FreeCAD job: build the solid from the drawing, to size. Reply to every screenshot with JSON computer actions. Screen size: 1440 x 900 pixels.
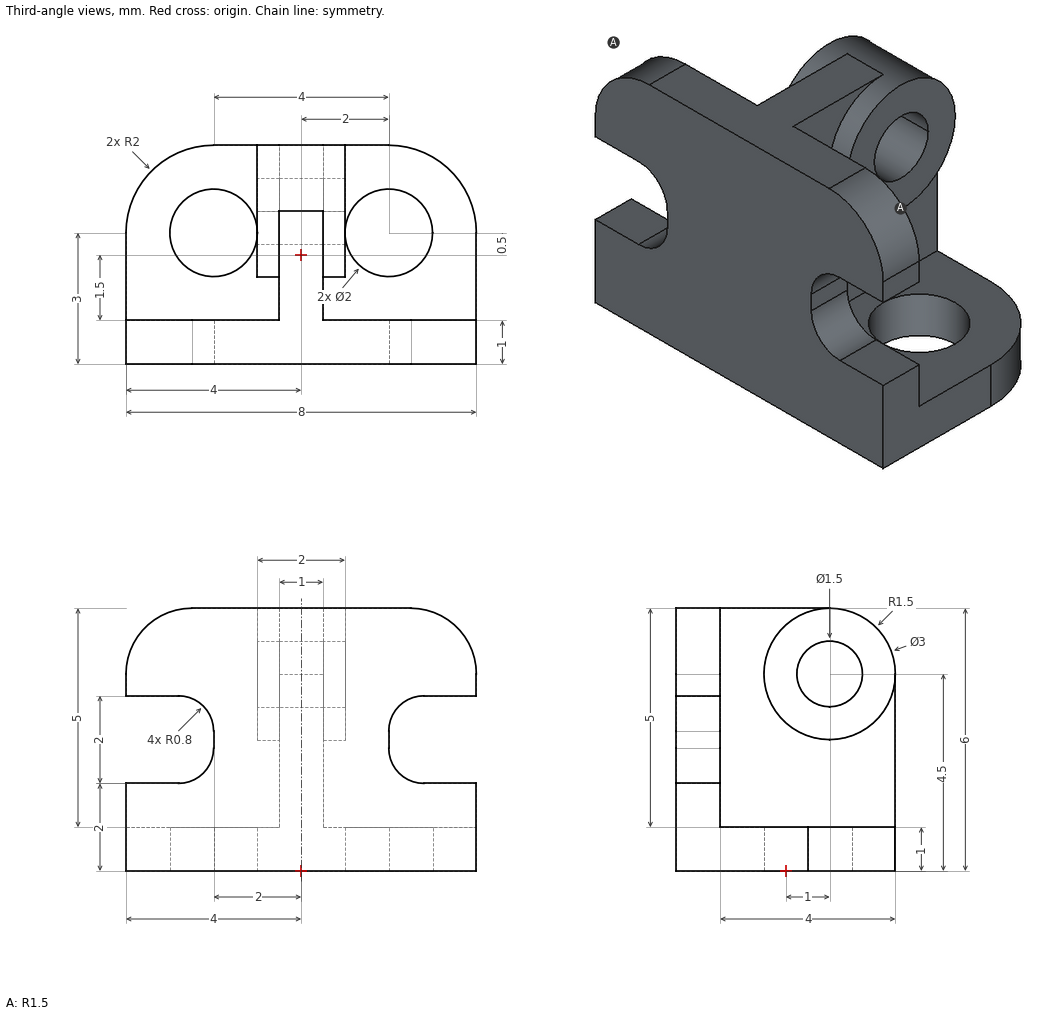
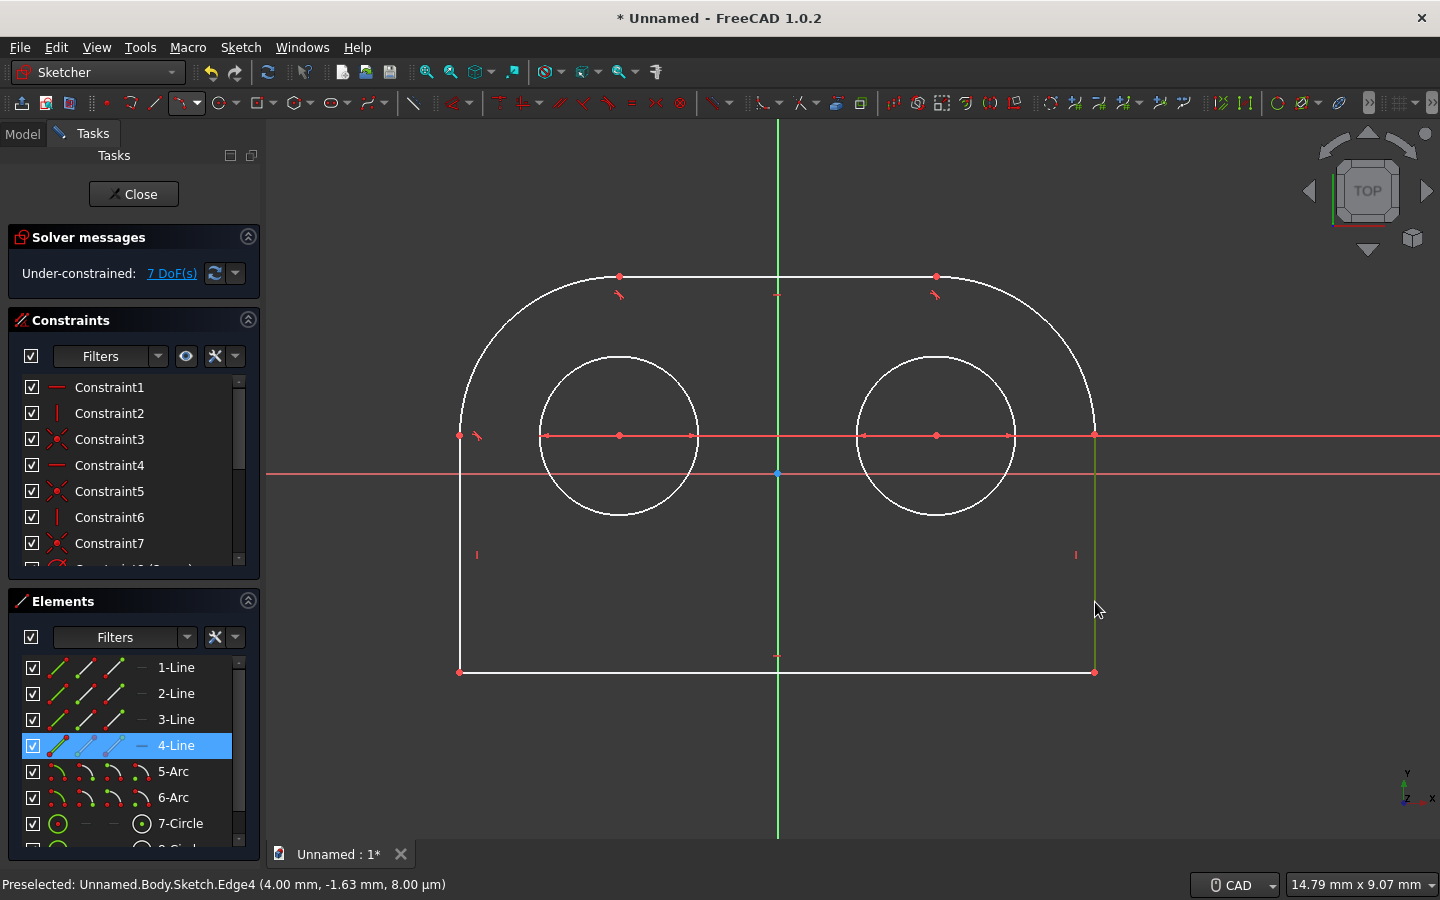
{"action": "left_click", "coordinate": [1077, 363]}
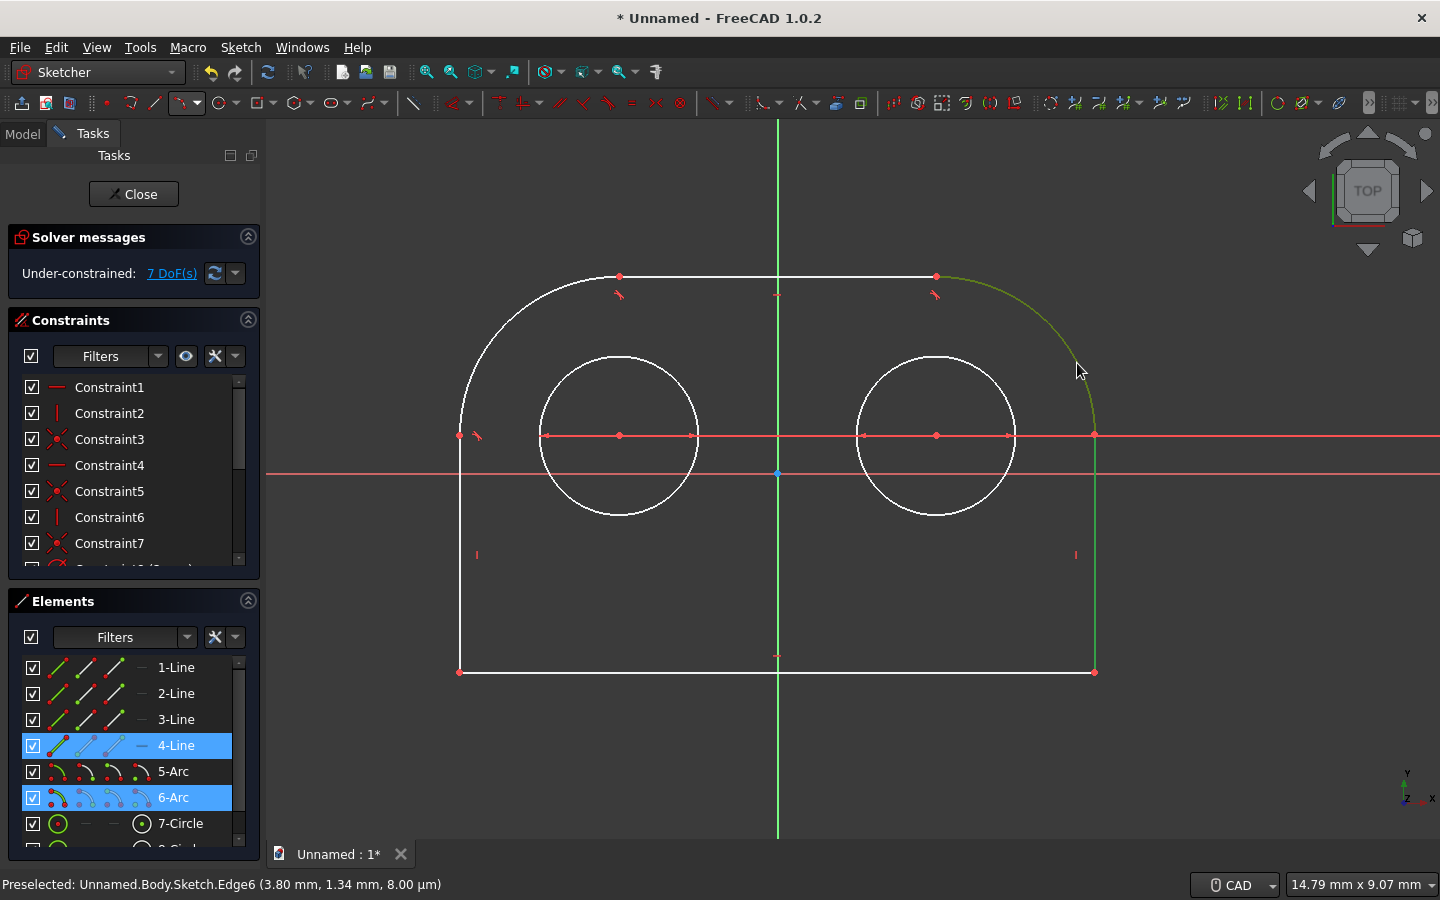
{"action": "key", "text": "t"}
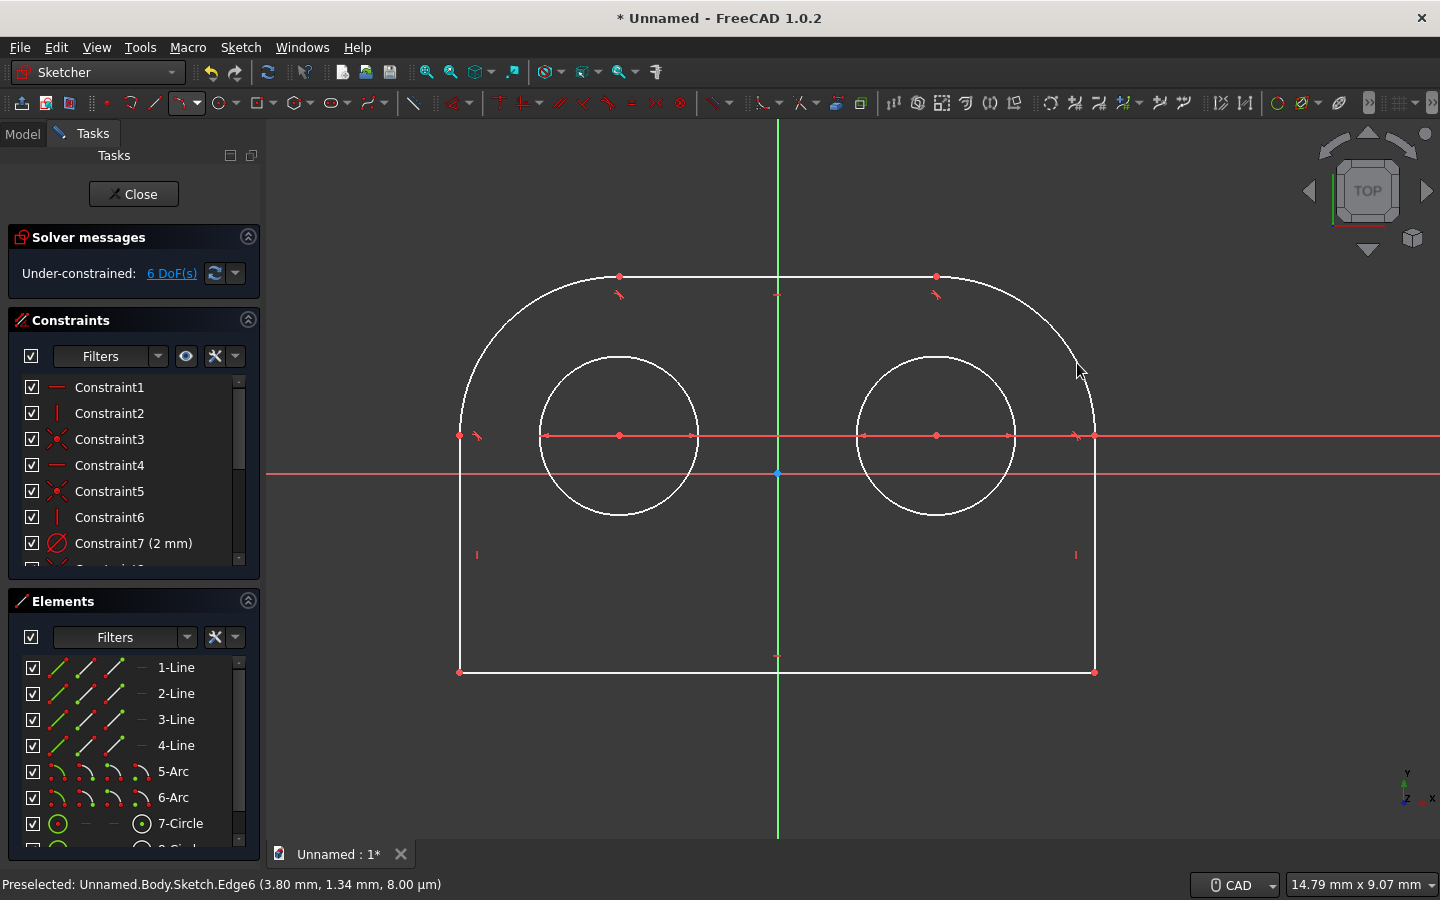
{"action": "left_click", "coordinate": [547, 294]}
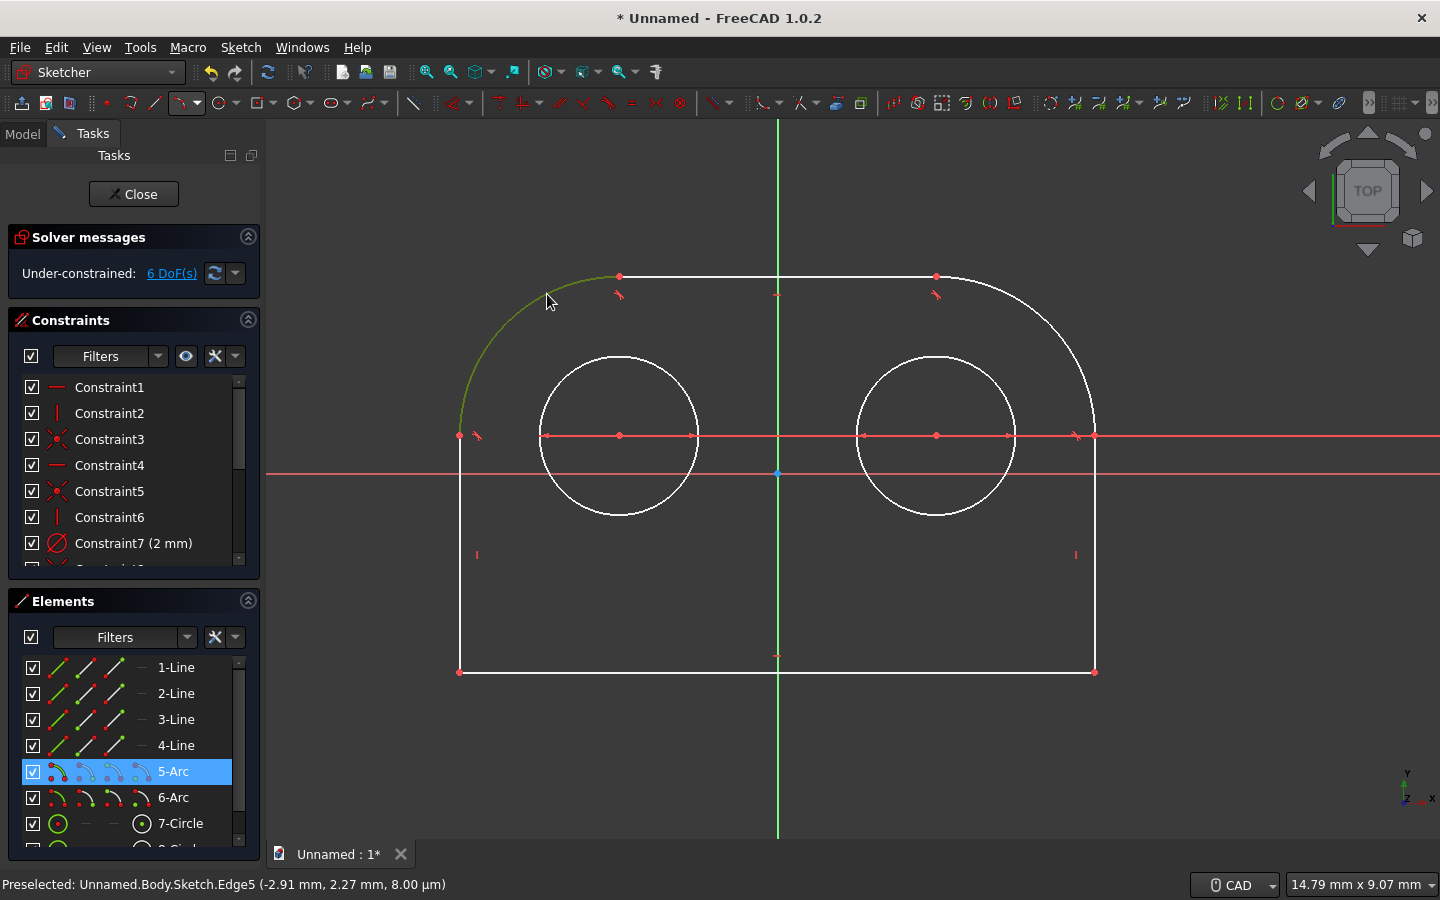
{"action": "left_click", "coordinate": [1078, 364]}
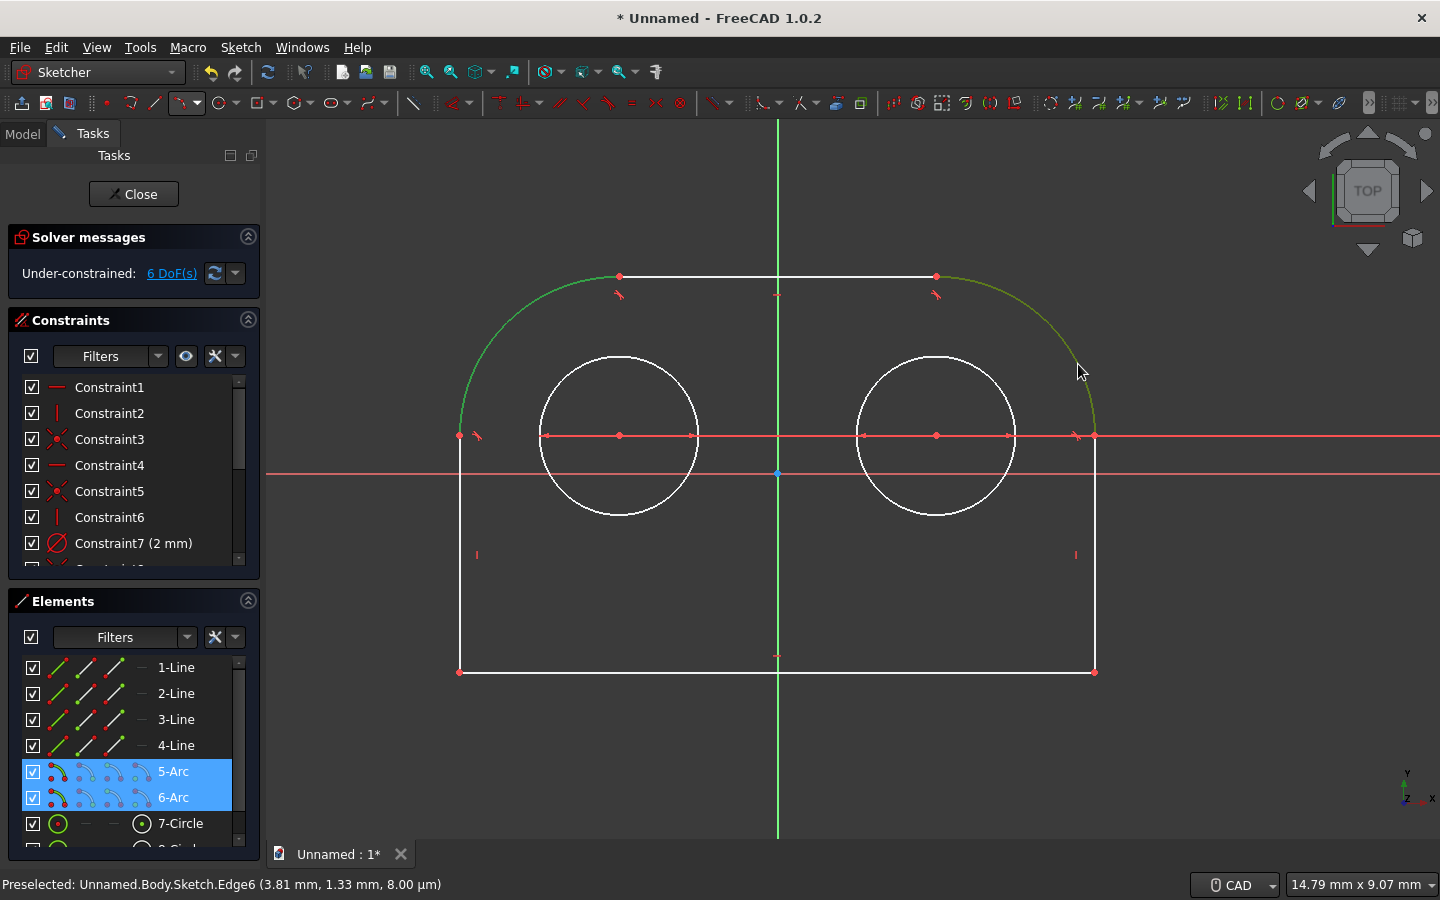
{"action": "left_click", "coordinate": [632, 104]}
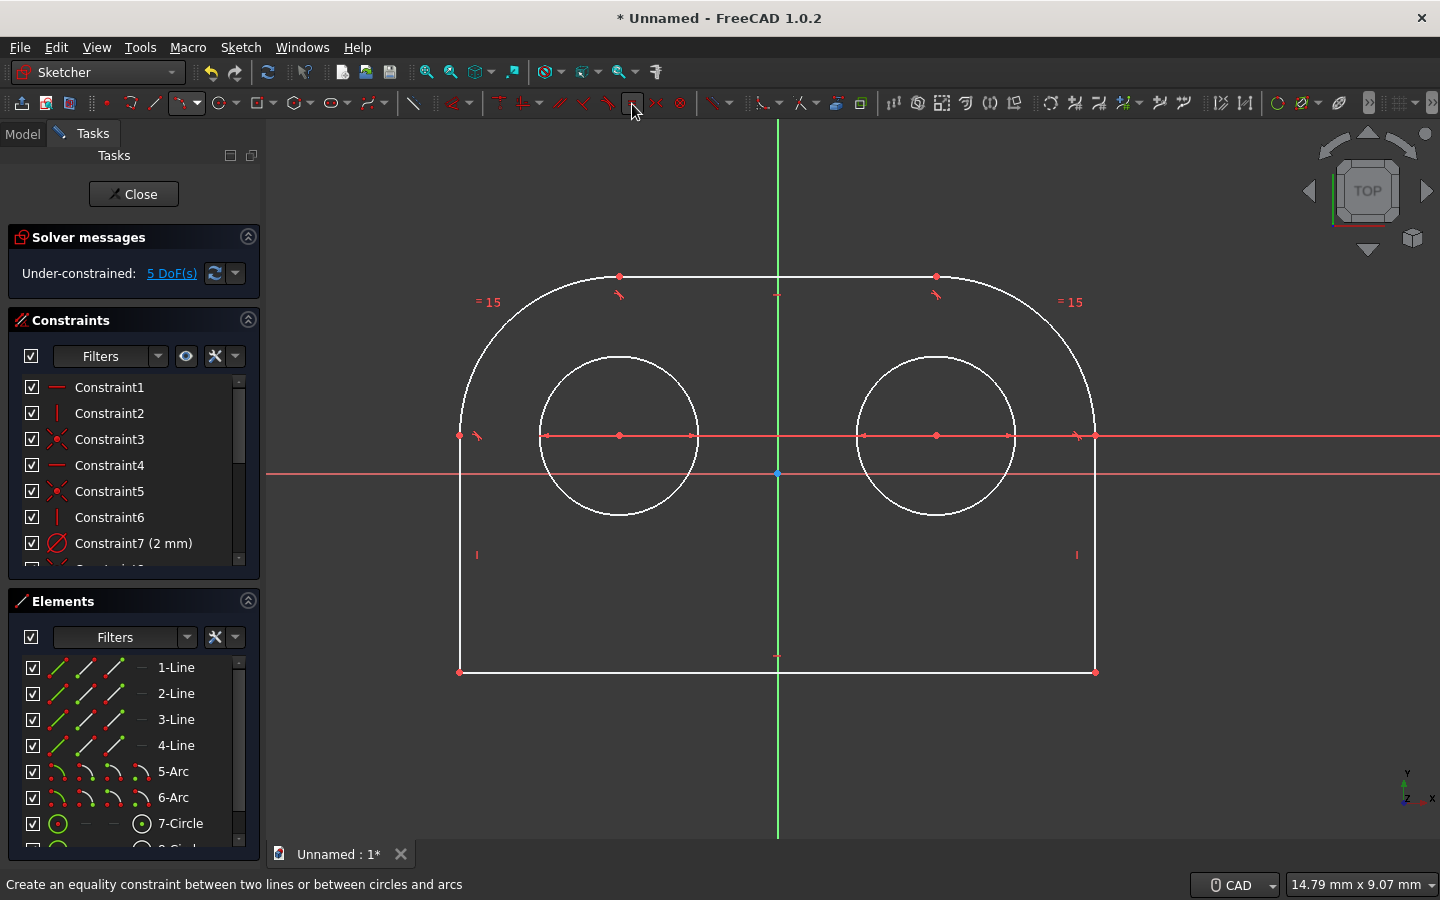
{"action": "left_click", "coordinate": [547, 294]}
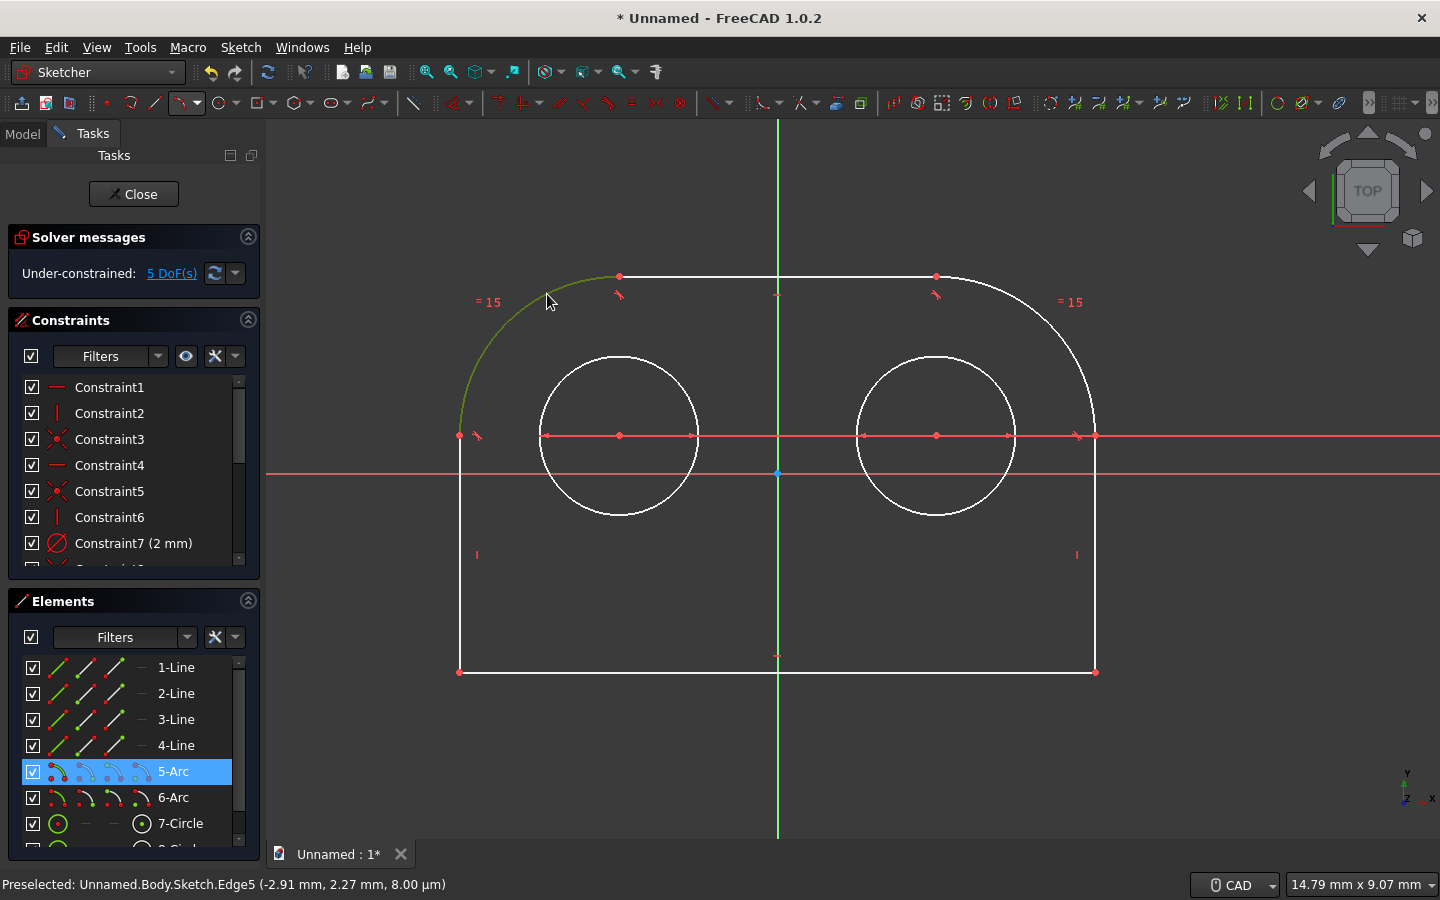
{"action": "left_click", "coordinate": [472, 104]}